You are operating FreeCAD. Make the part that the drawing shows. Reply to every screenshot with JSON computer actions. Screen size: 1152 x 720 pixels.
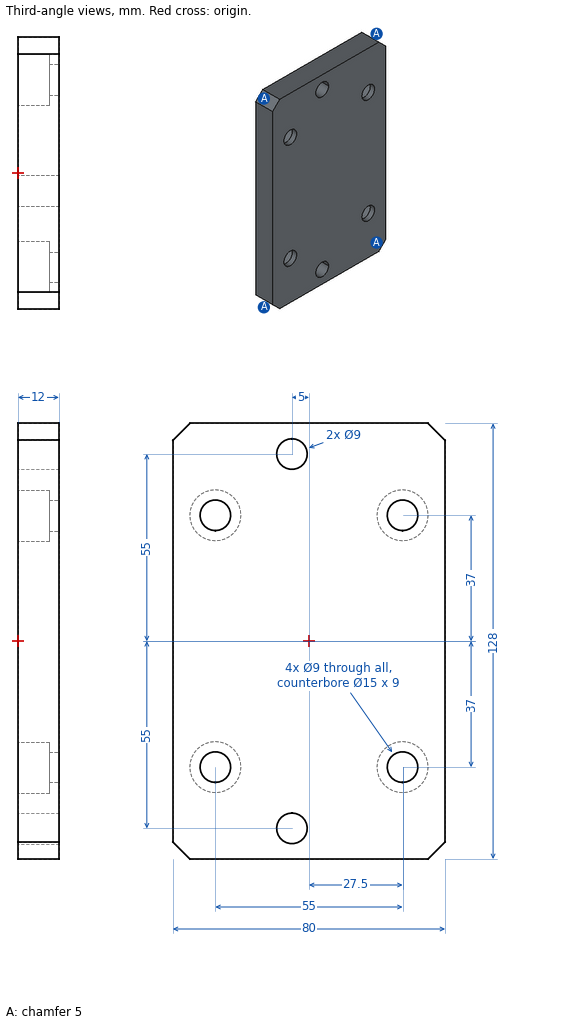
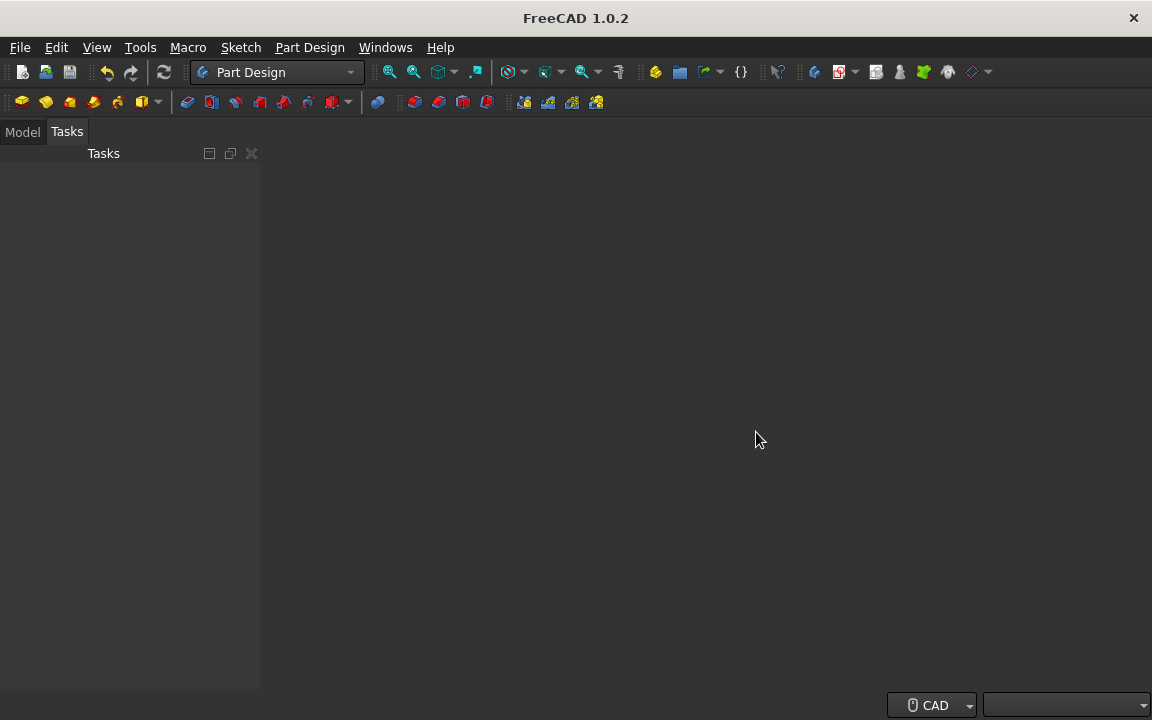
{"action": "left_click", "coordinate": [22, 72]}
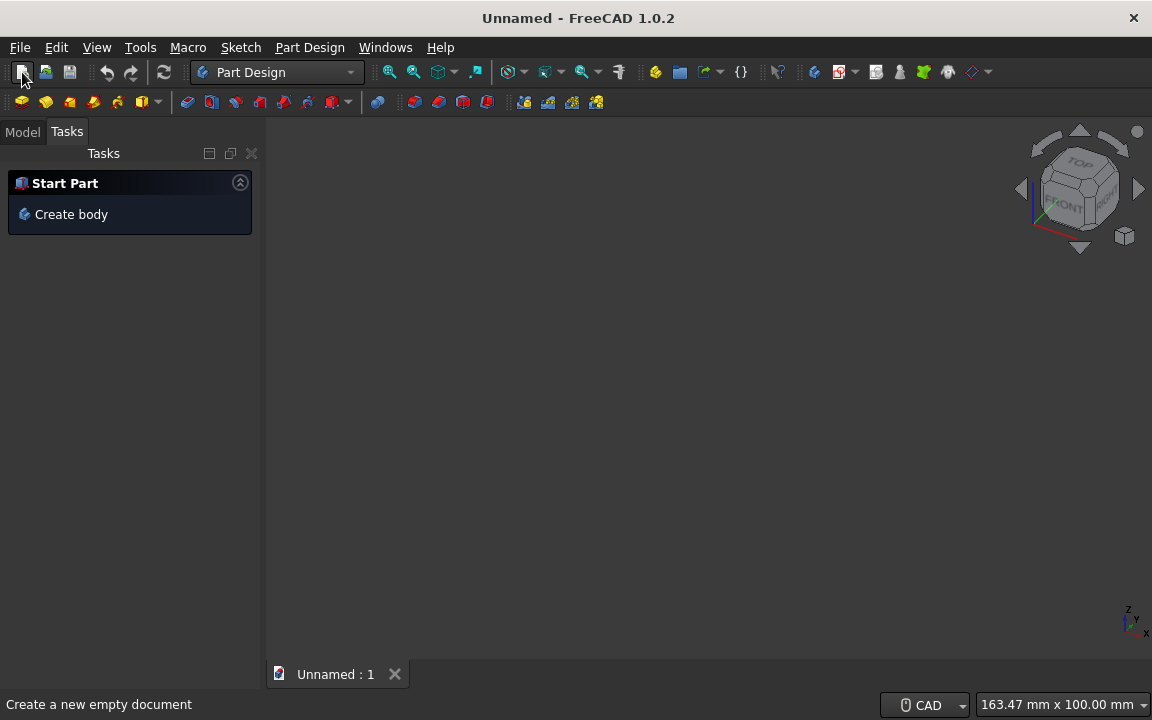
{"action": "left_click", "coordinate": [840, 72]}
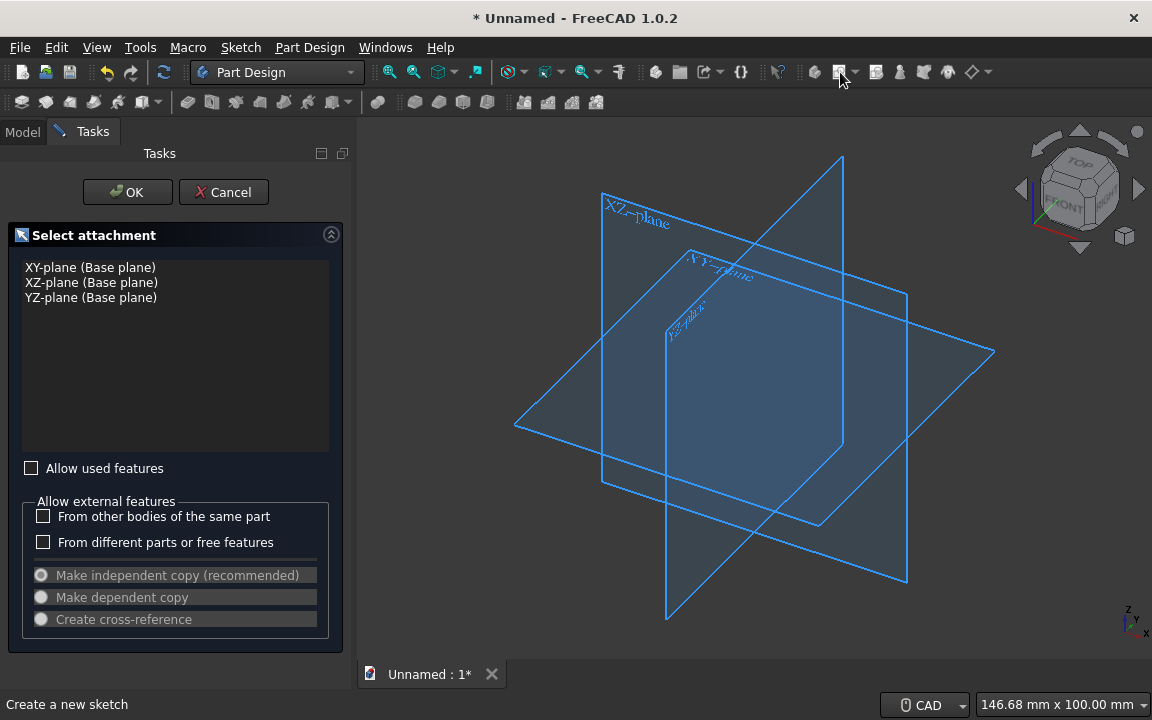
{"action": "left_click", "coordinate": [82, 298]}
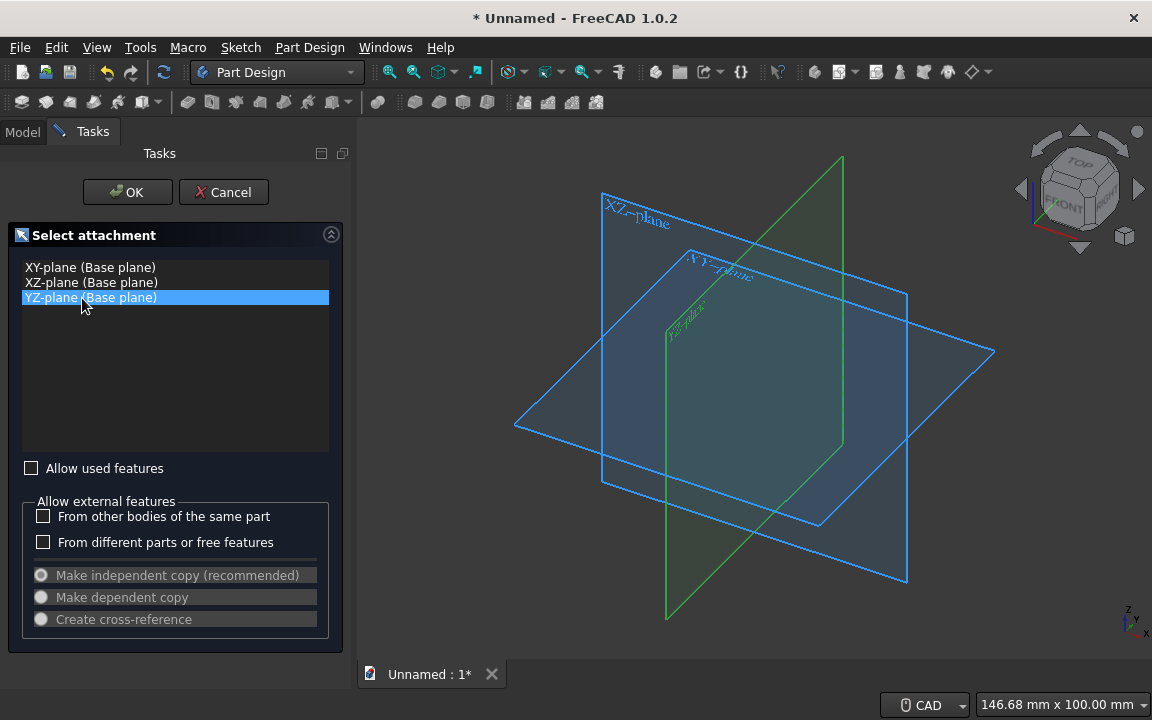
{"action": "left_click", "coordinate": [128, 192]}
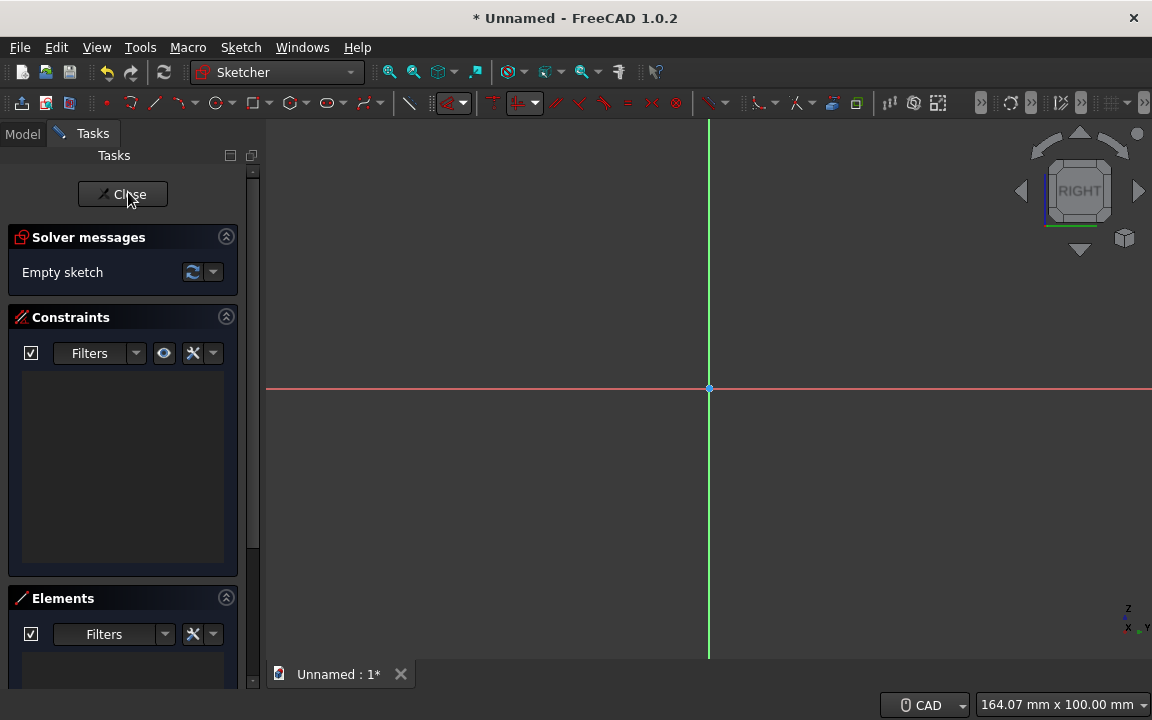
{"action": "scroll", "coordinate": [585, 389], "scroll_direction": "down", "scroll_amount": 4}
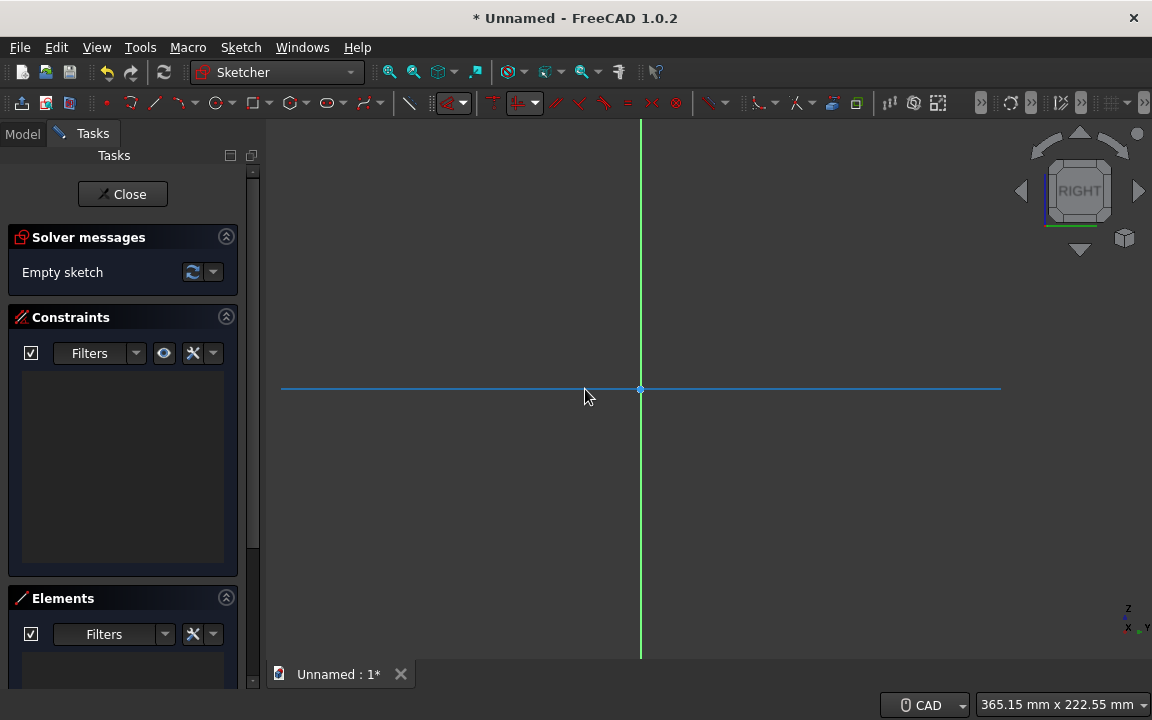
{"action": "left_click", "coordinate": [272, 104]}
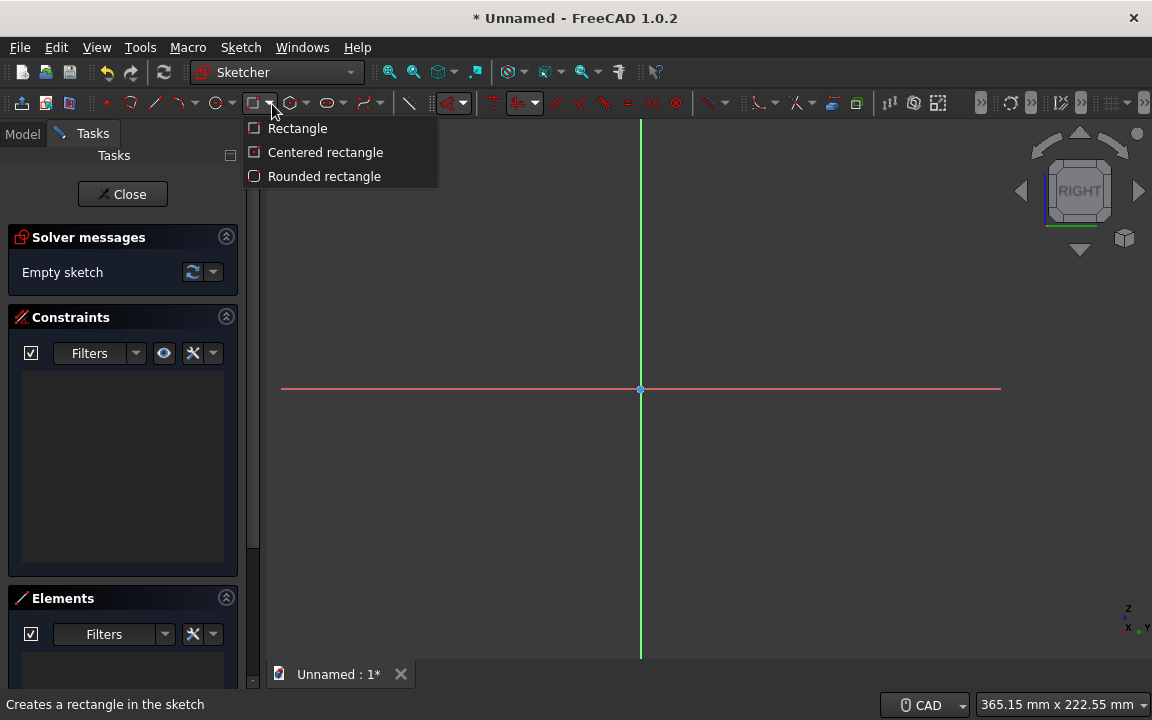
{"action": "left_click", "coordinate": [340, 152]}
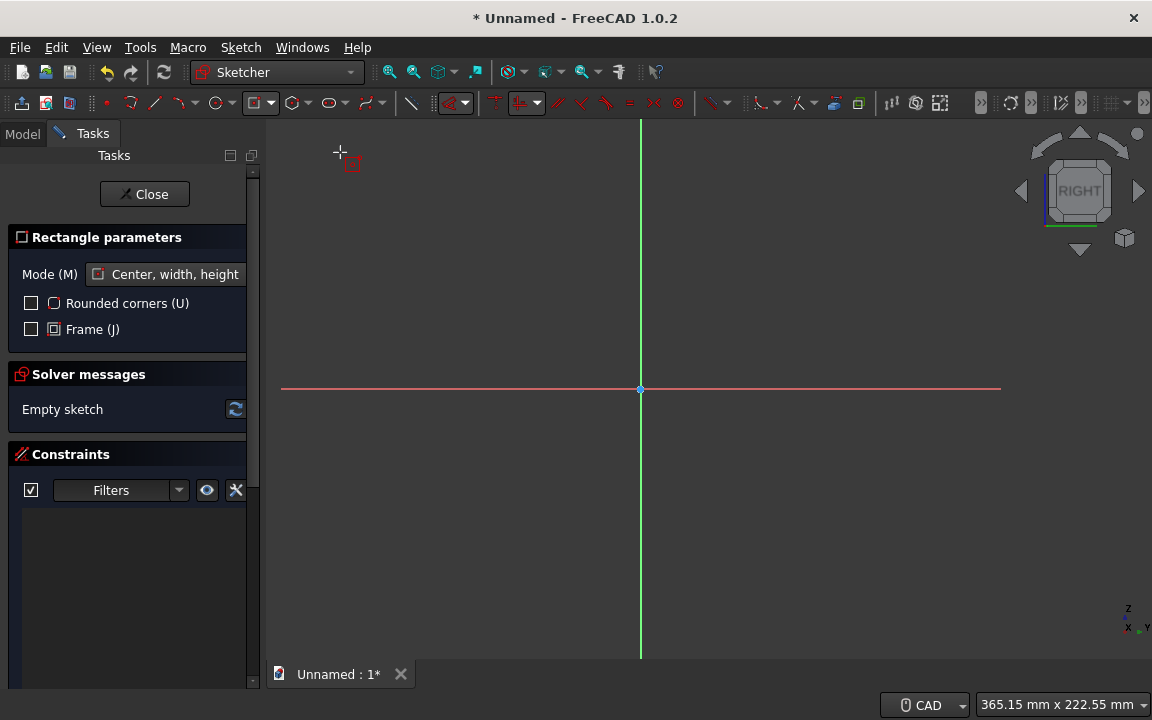
{"action": "left_click", "coordinate": [641, 389]}
{"action": "left_click", "coordinate": [738, 234]}
{"action": "key", "text": "Escape"}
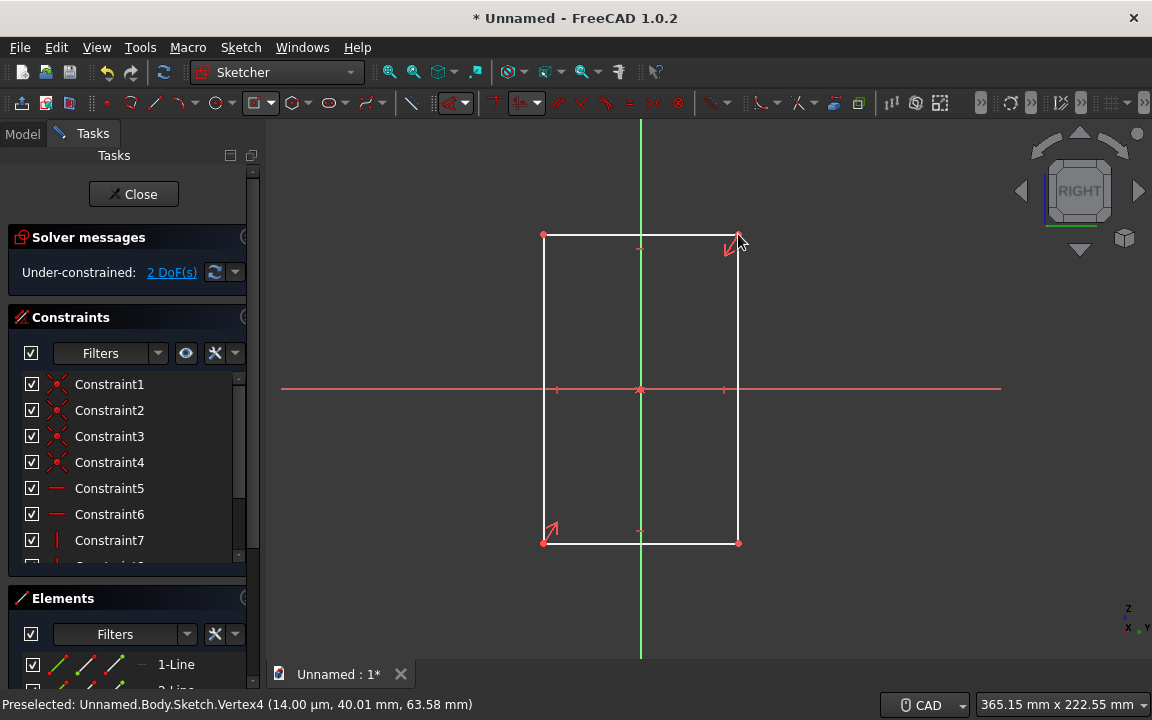
{"action": "left_click", "coordinate": [450, 104]}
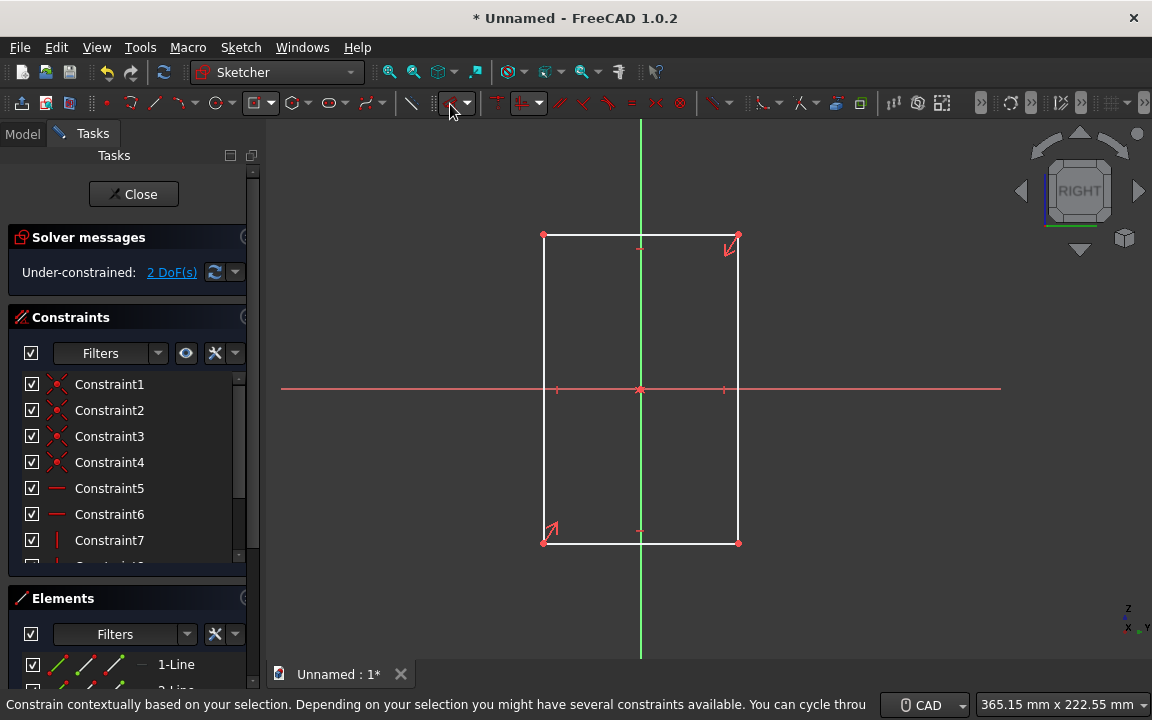
{"action": "left_click", "coordinate": [602, 544]}
{"action": "left_click", "coordinate": [596, 578]}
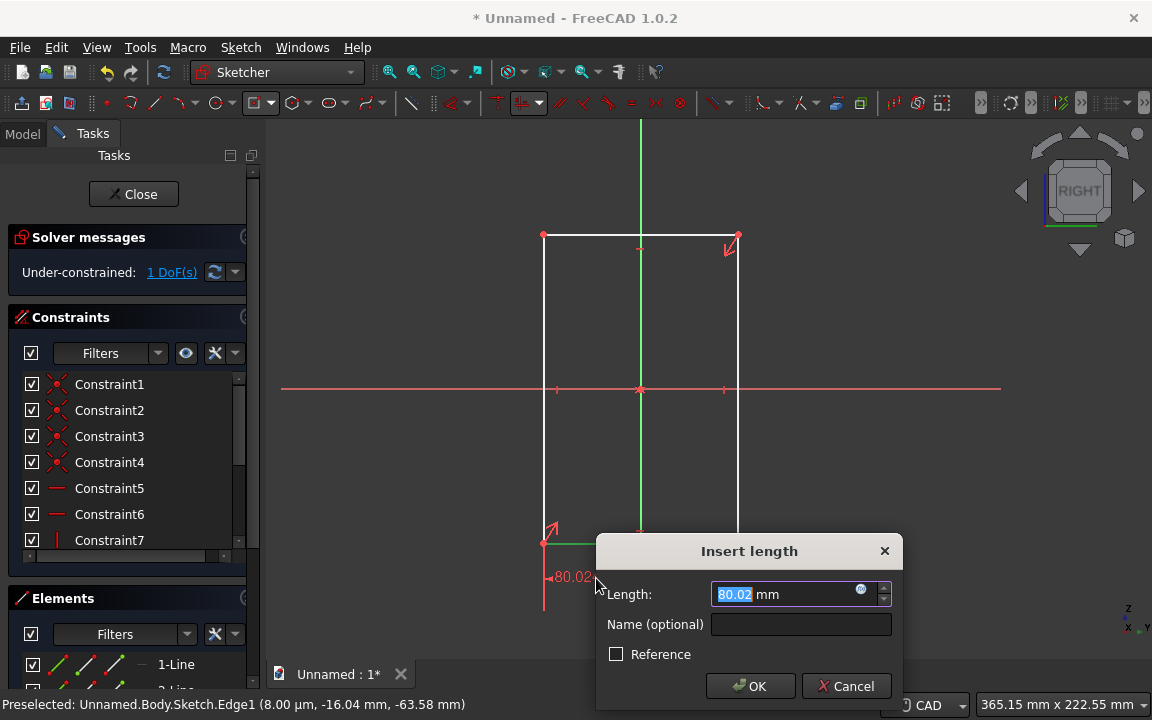
{"action": "type", "text": "80"}
{"action": "key", "text": "Return"}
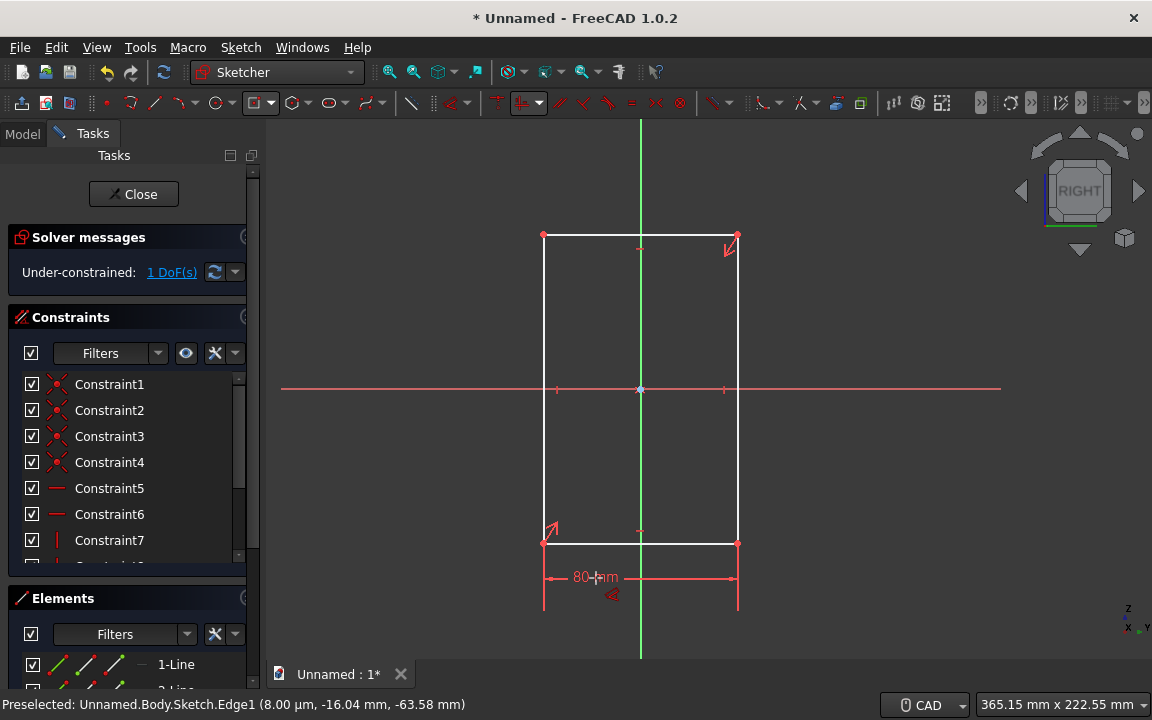
{"action": "left_click", "coordinate": [738, 451]}
{"action": "left_click", "coordinate": [772, 318]}